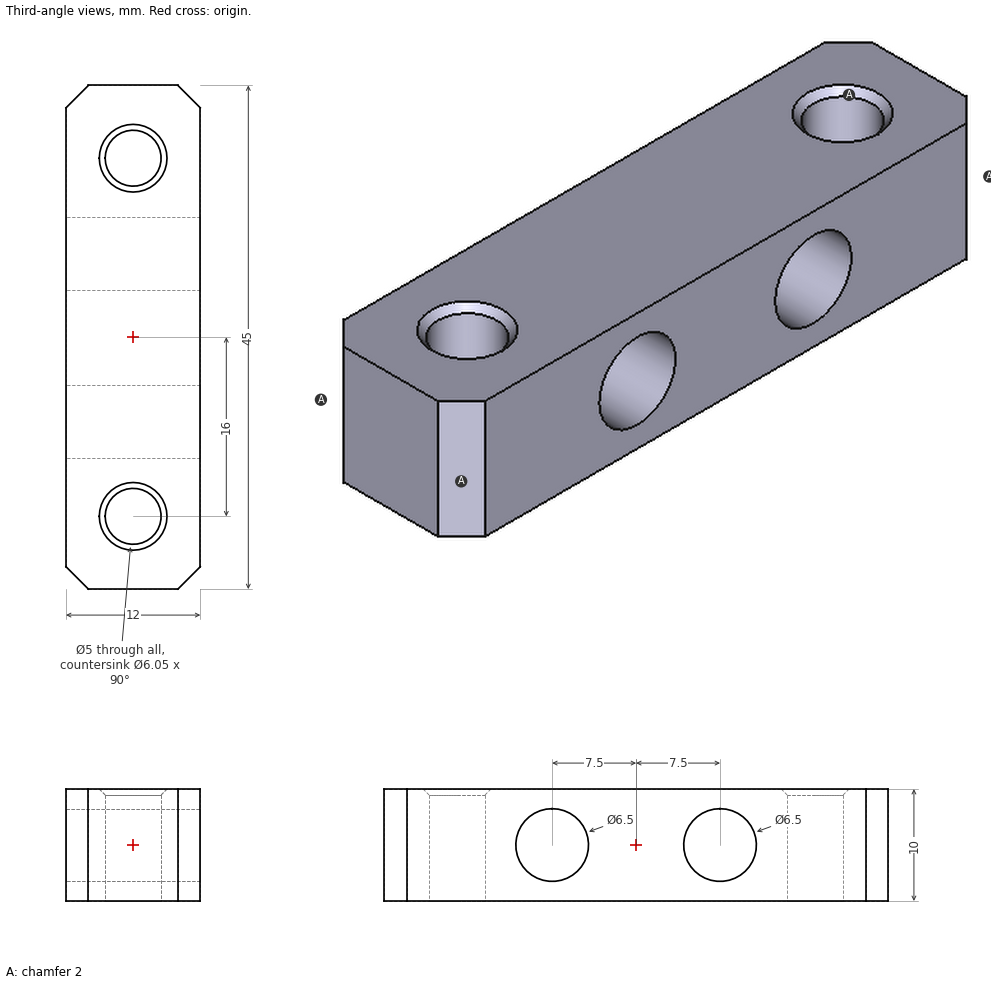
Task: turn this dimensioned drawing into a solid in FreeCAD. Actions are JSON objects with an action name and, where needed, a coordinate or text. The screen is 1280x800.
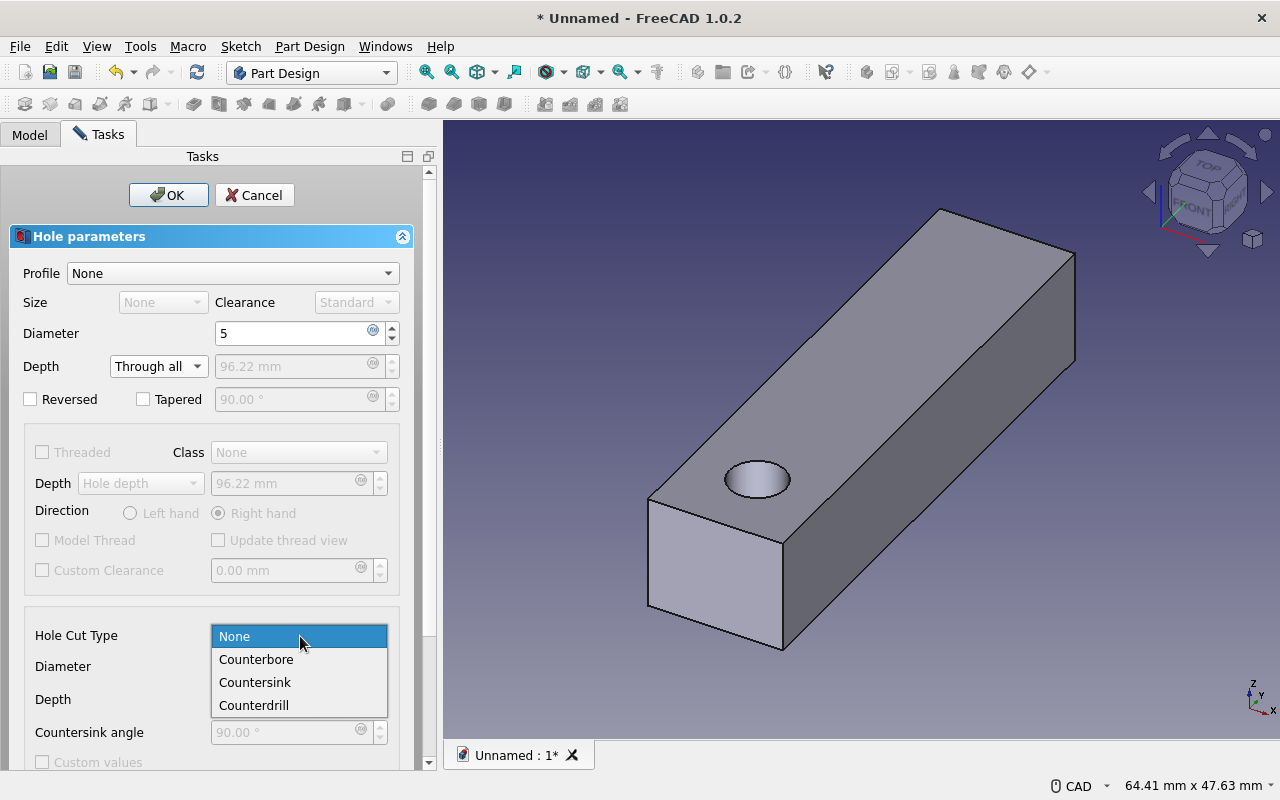
{"action": "left_click", "coordinate": [298, 682]}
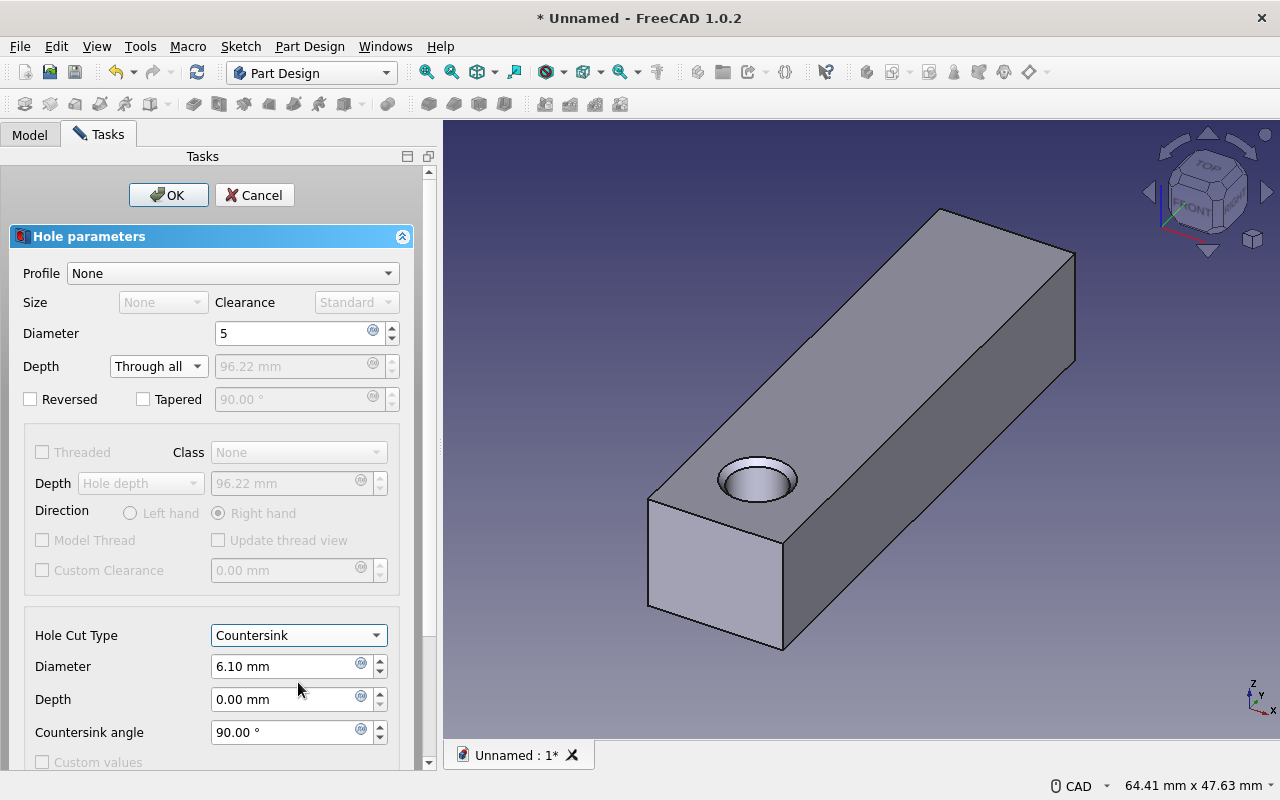
{"action": "triple_click", "coordinate": [292, 666]}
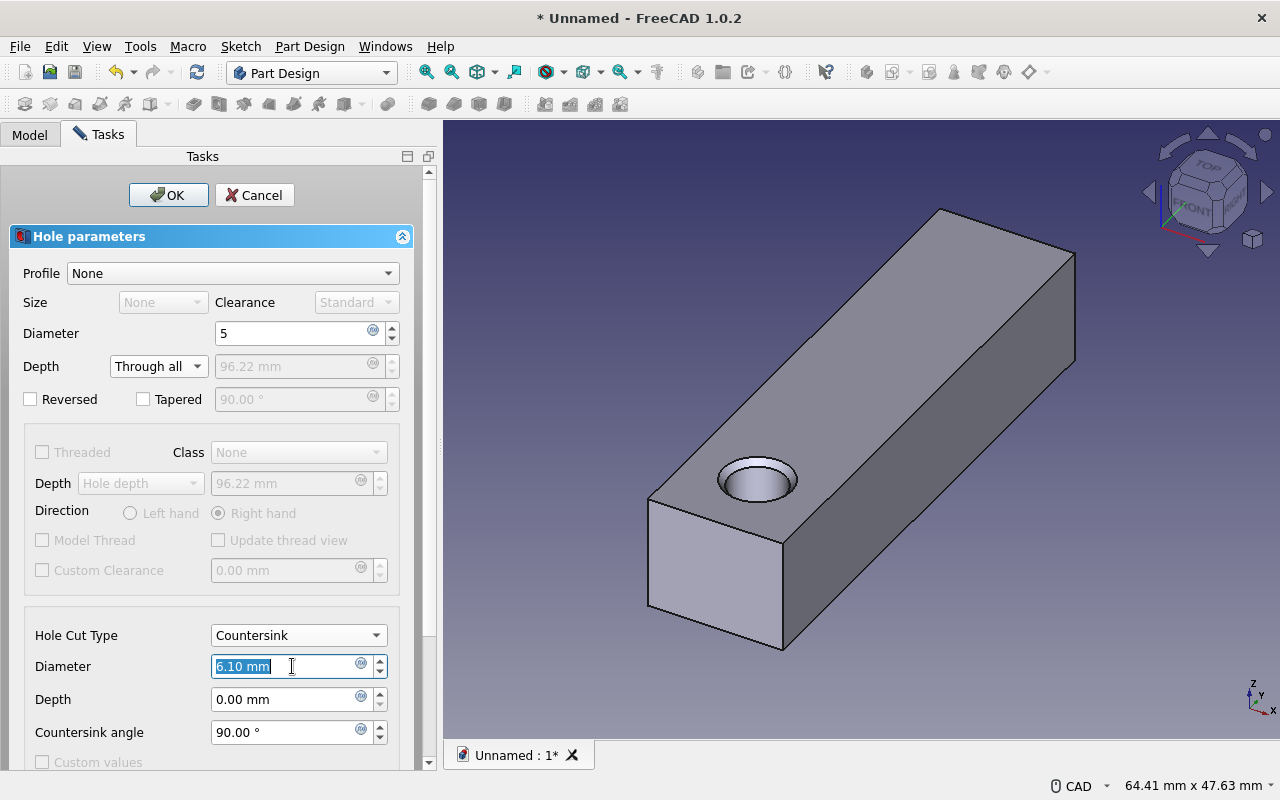
{"action": "type", "text": "6.05"}
{"action": "key", "text": "Tab"}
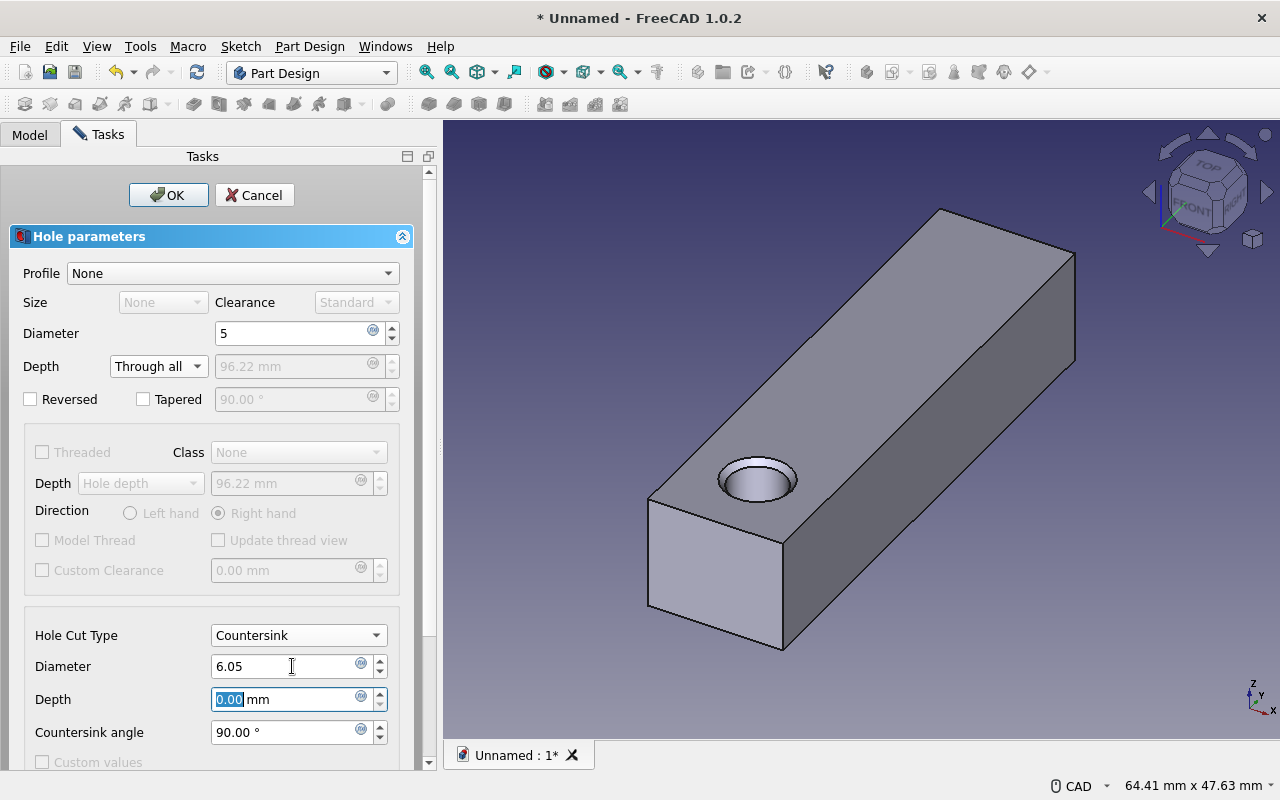
{"action": "left_click", "coordinate": [169, 195]}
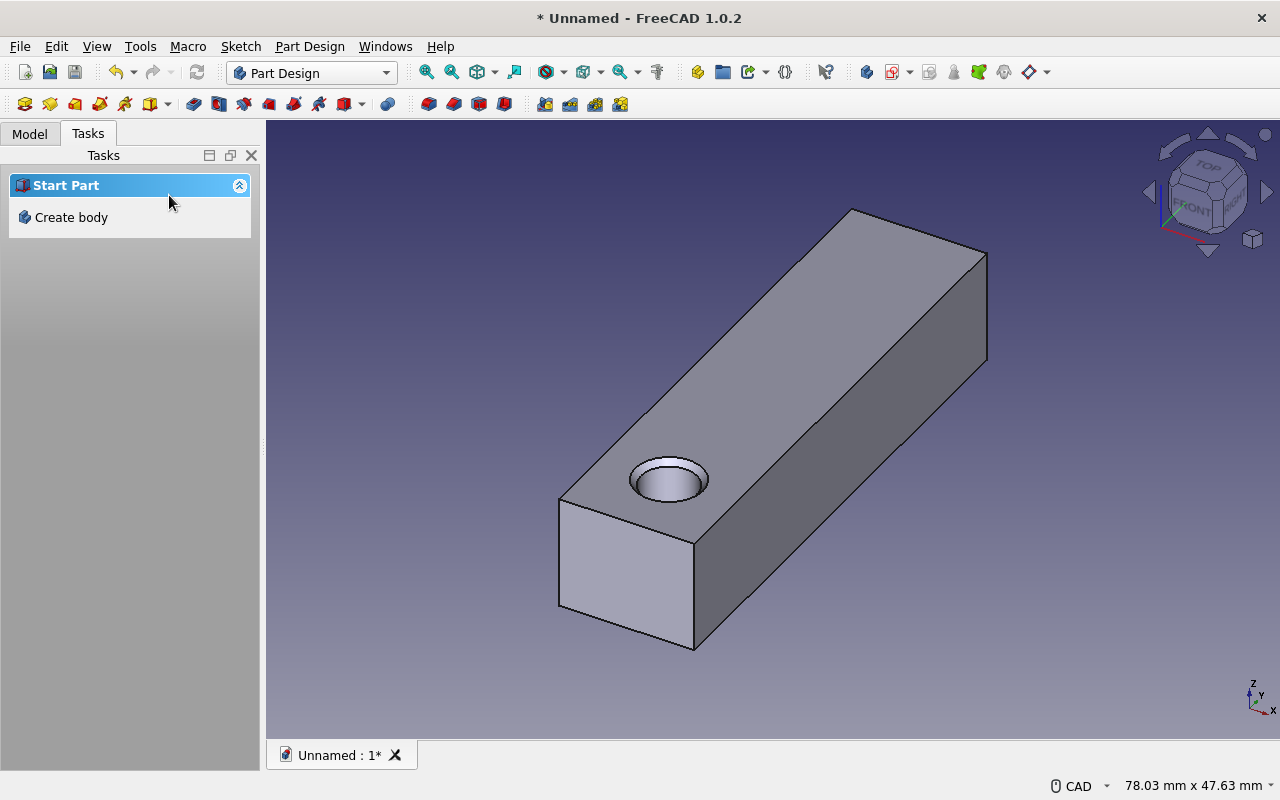
{"action": "key", "text": "6"}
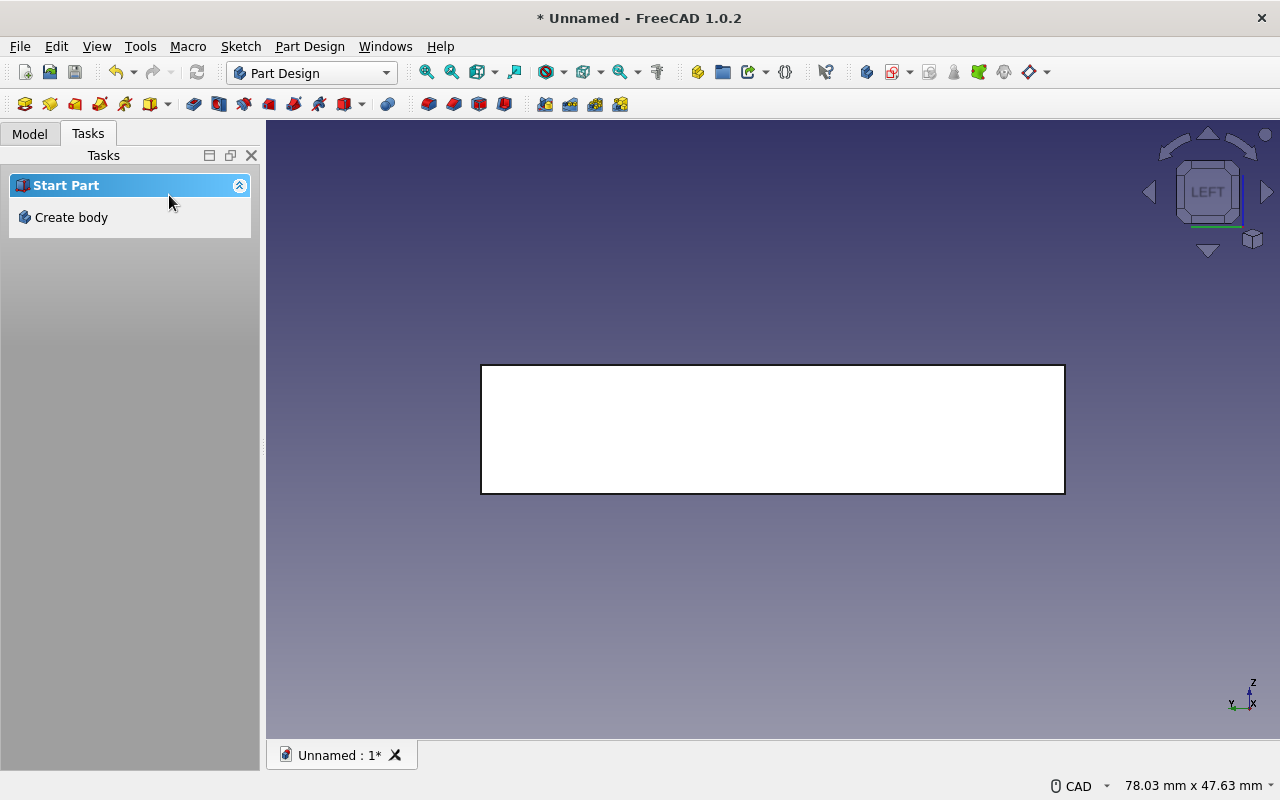
{"action": "left_click", "coordinate": [606, 428]}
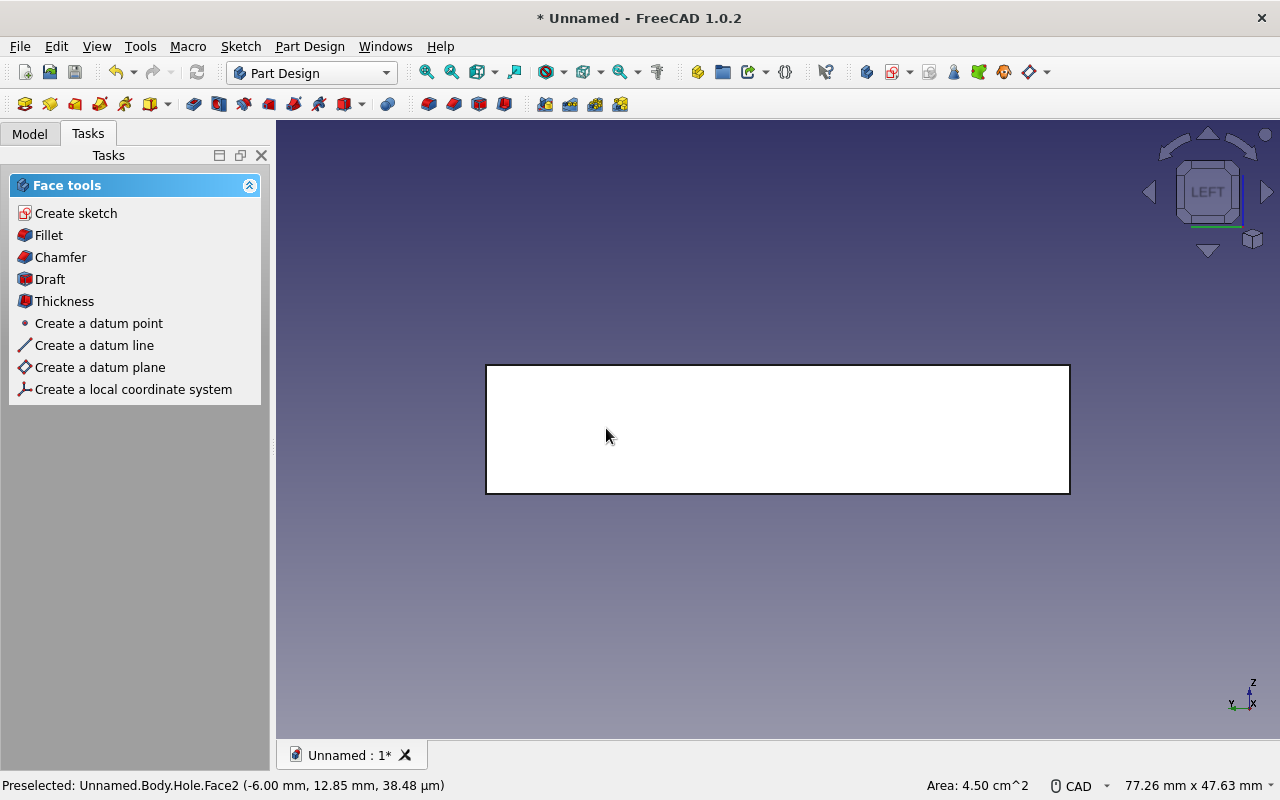
{"action": "left_click", "coordinate": [892, 72]}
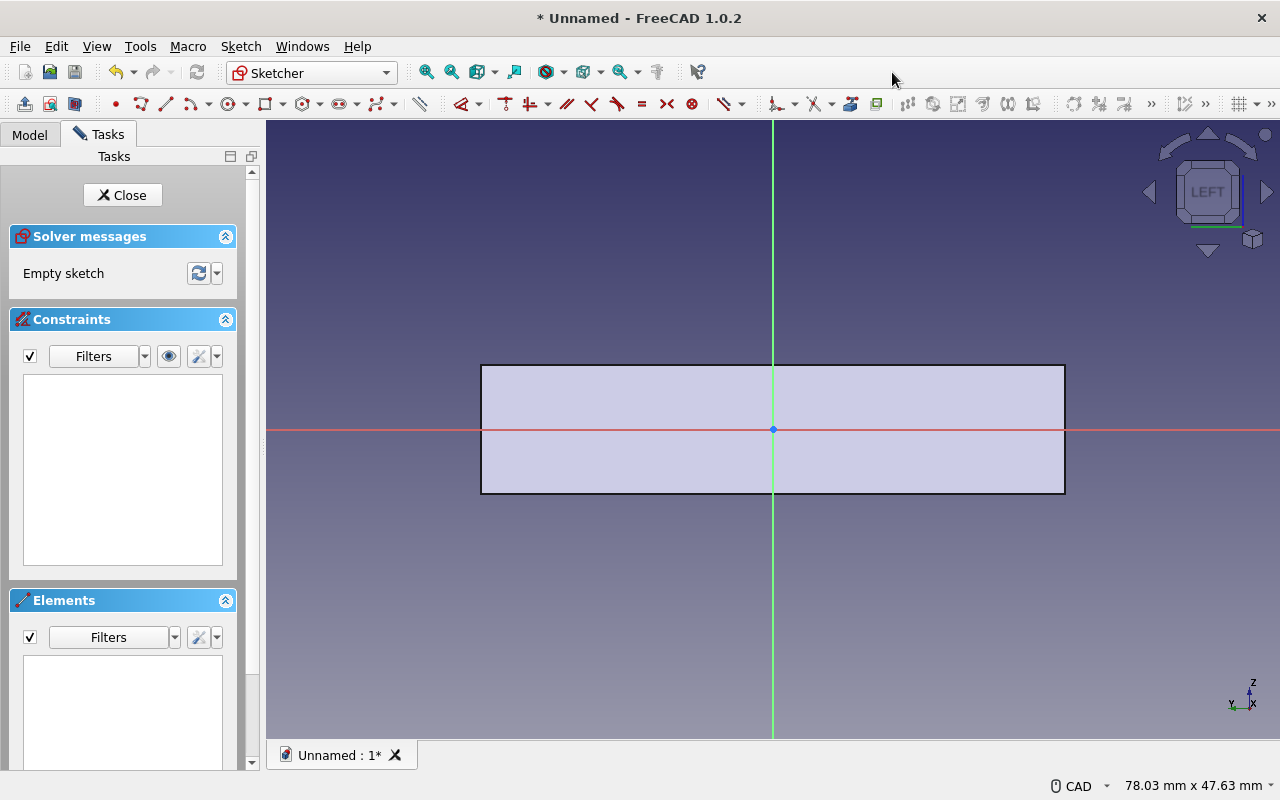
{"action": "scroll", "coordinate": [703, 430], "scroll_direction": "up", "scroll_amount": 7}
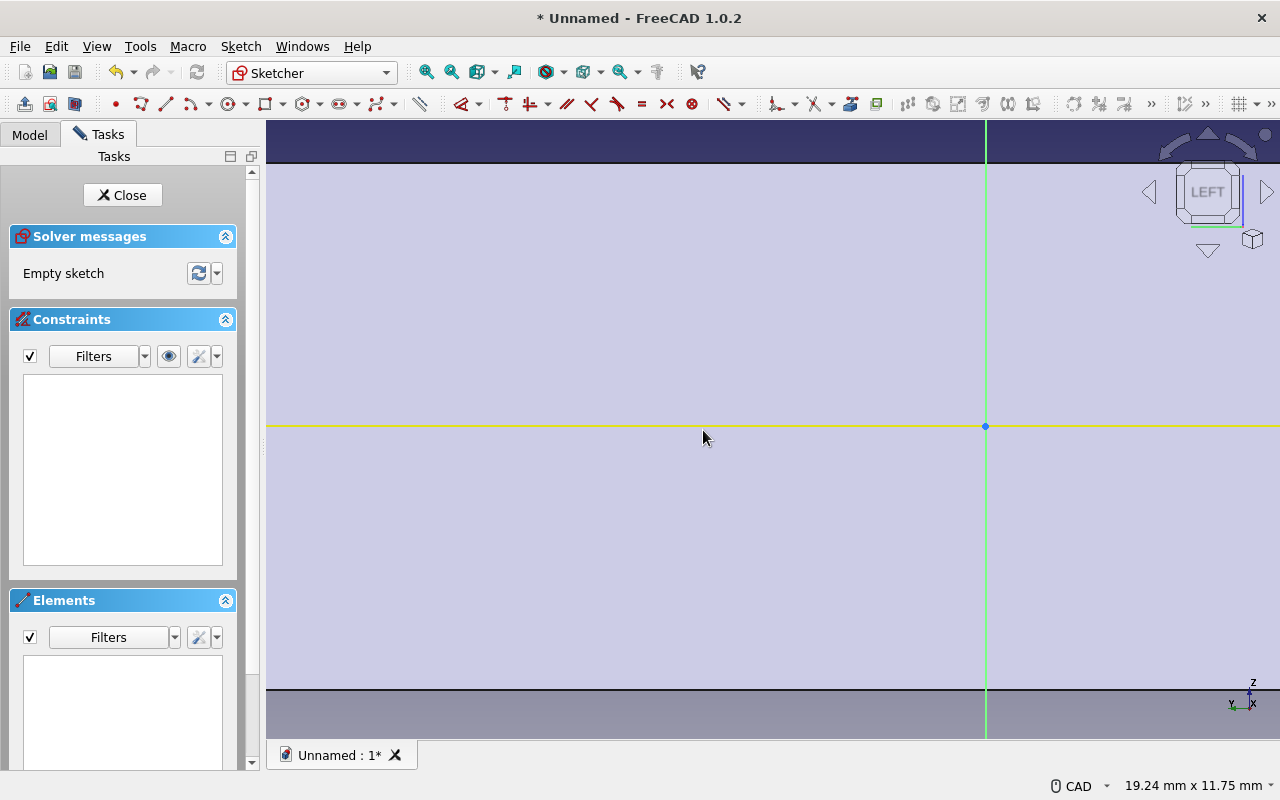
{"action": "left_click", "coordinate": [228, 104]}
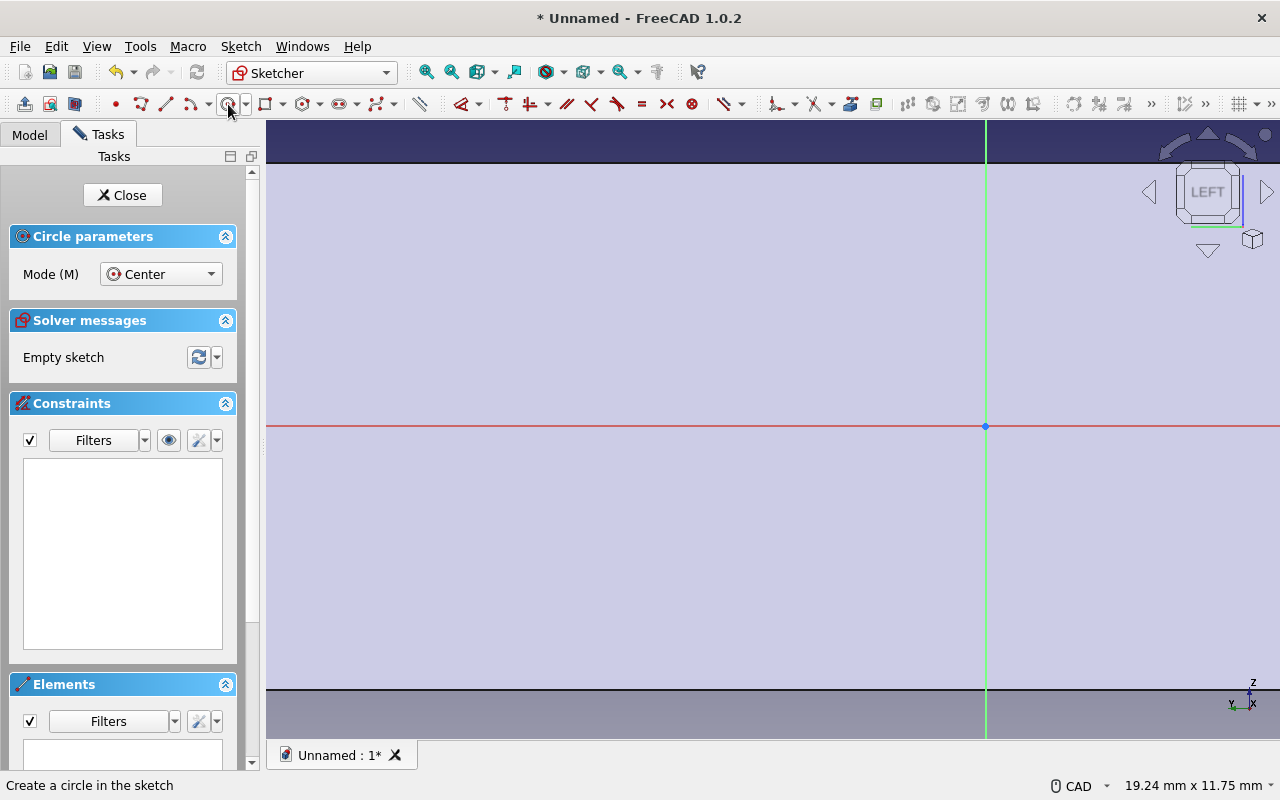
{"action": "left_click", "coordinate": [590, 426]}
{"action": "mouse_move", "coordinate": [711, 305]}